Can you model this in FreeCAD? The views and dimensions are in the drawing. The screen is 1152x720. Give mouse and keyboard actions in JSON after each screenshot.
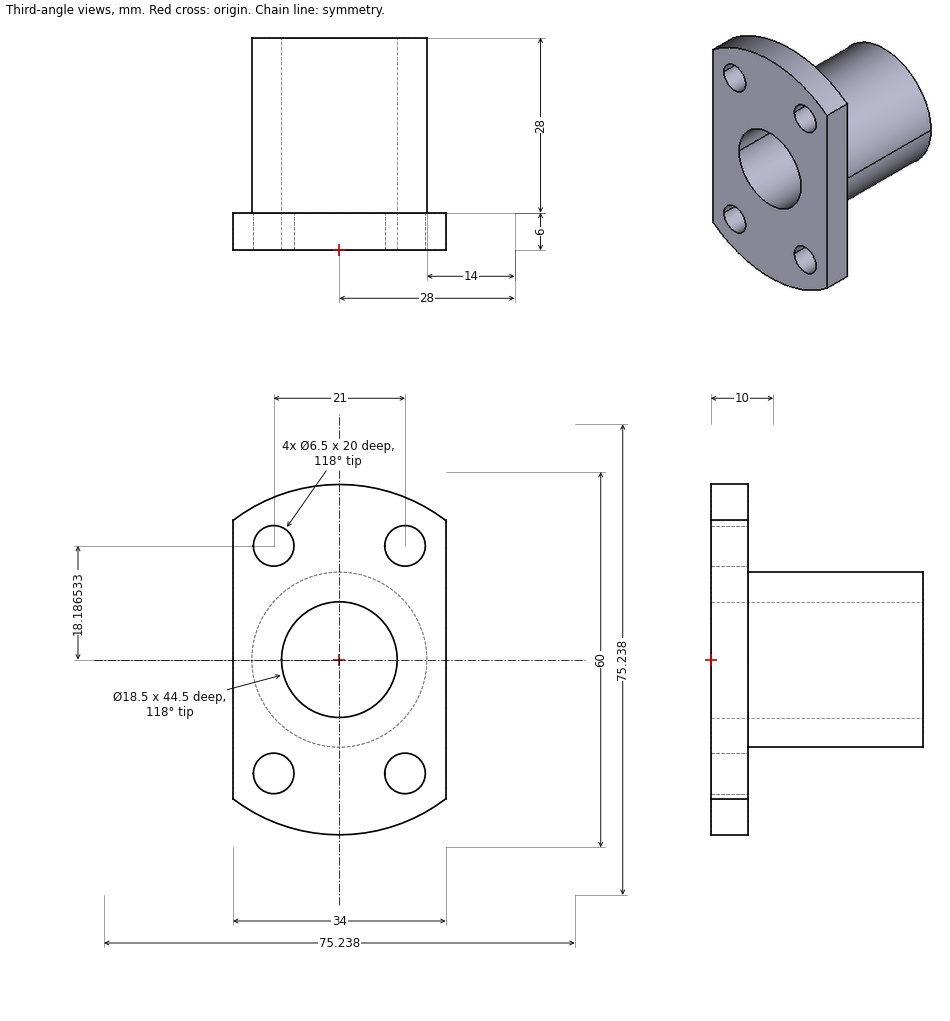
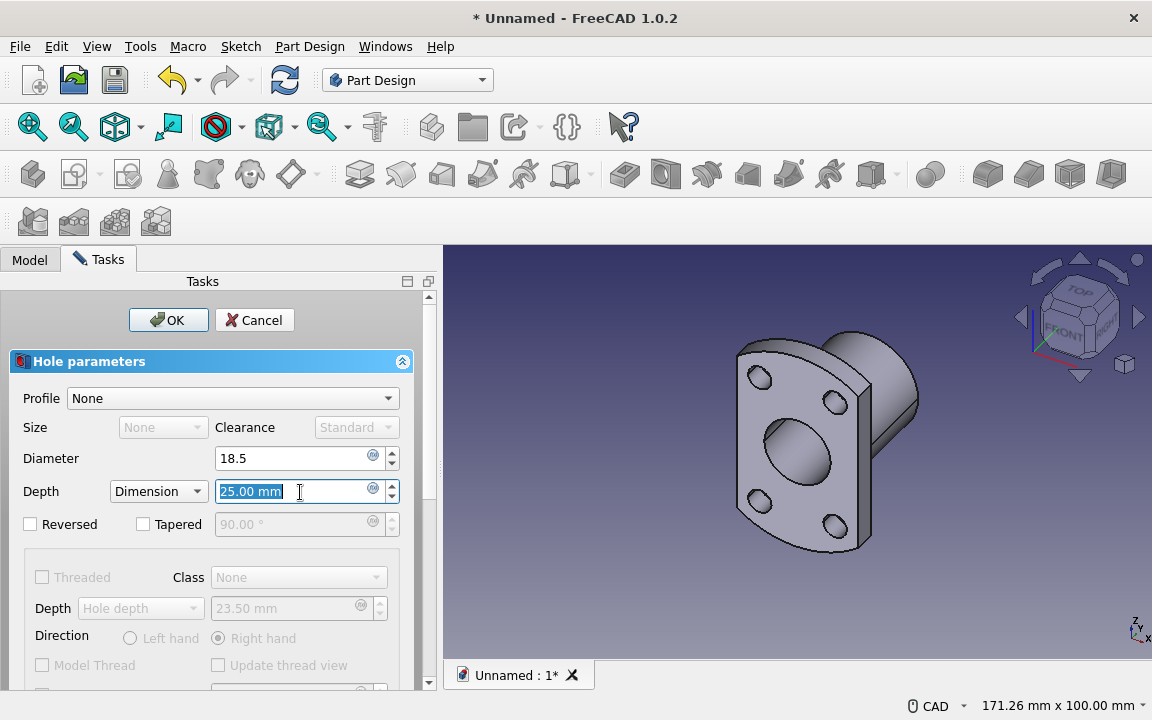
{"action": "type", "text": "44.5"}
{"action": "key", "text": "Tab"}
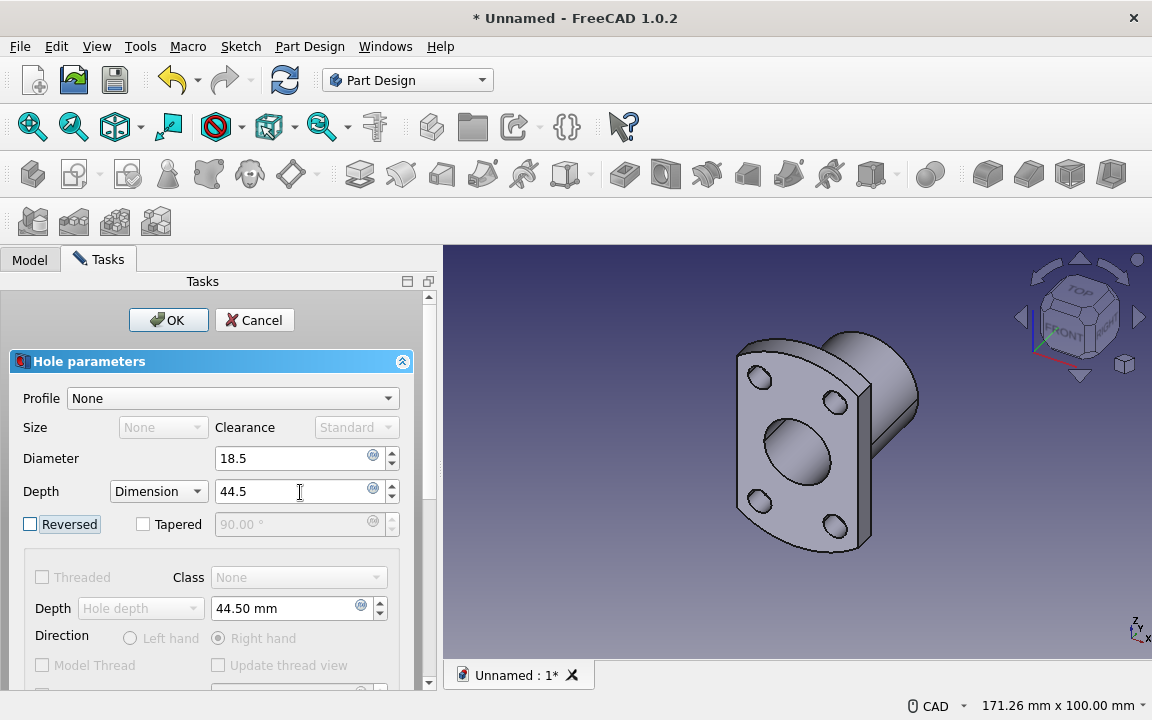
{"action": "left_click", "coordinate": [169, 320]}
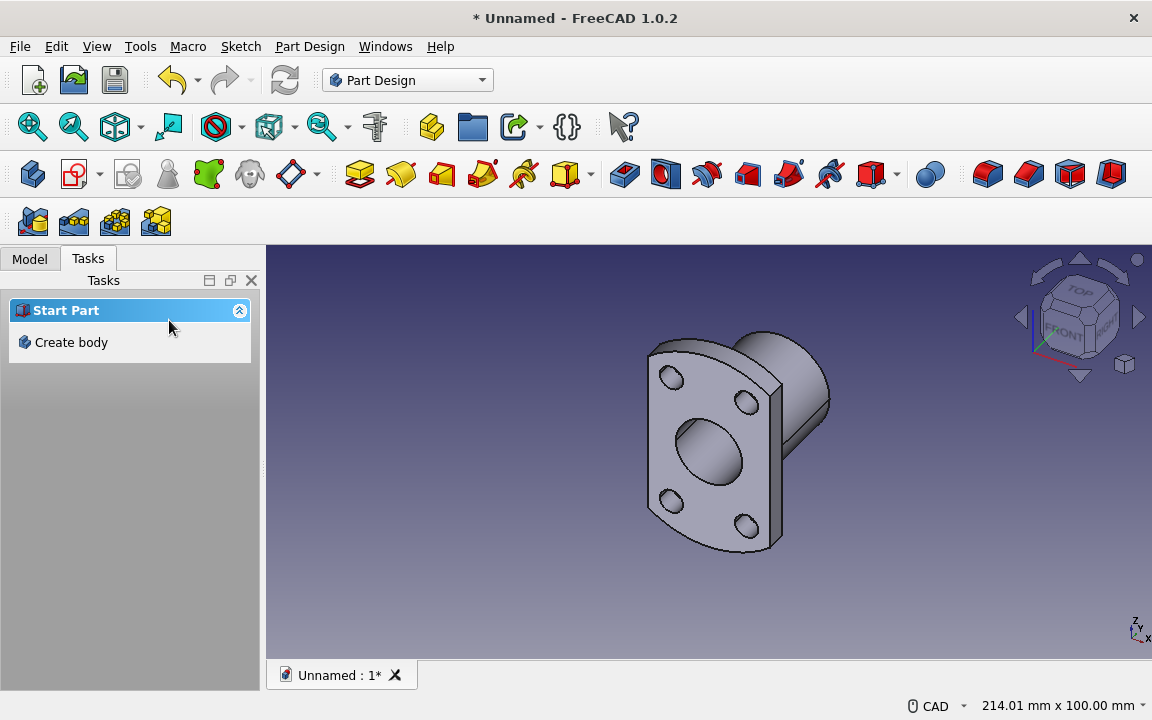
{"action": "key", "text": "0"}